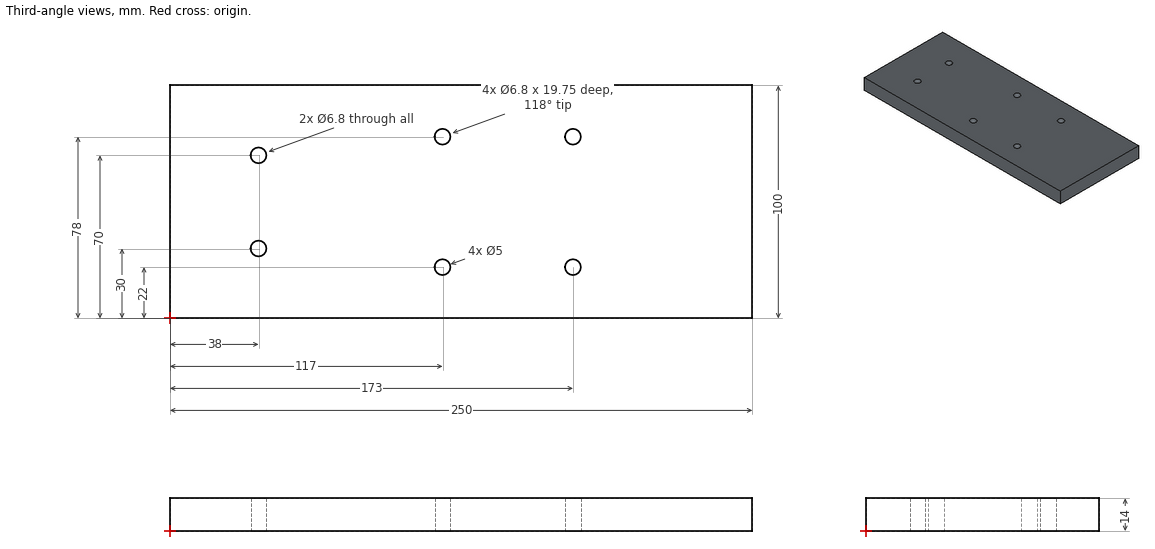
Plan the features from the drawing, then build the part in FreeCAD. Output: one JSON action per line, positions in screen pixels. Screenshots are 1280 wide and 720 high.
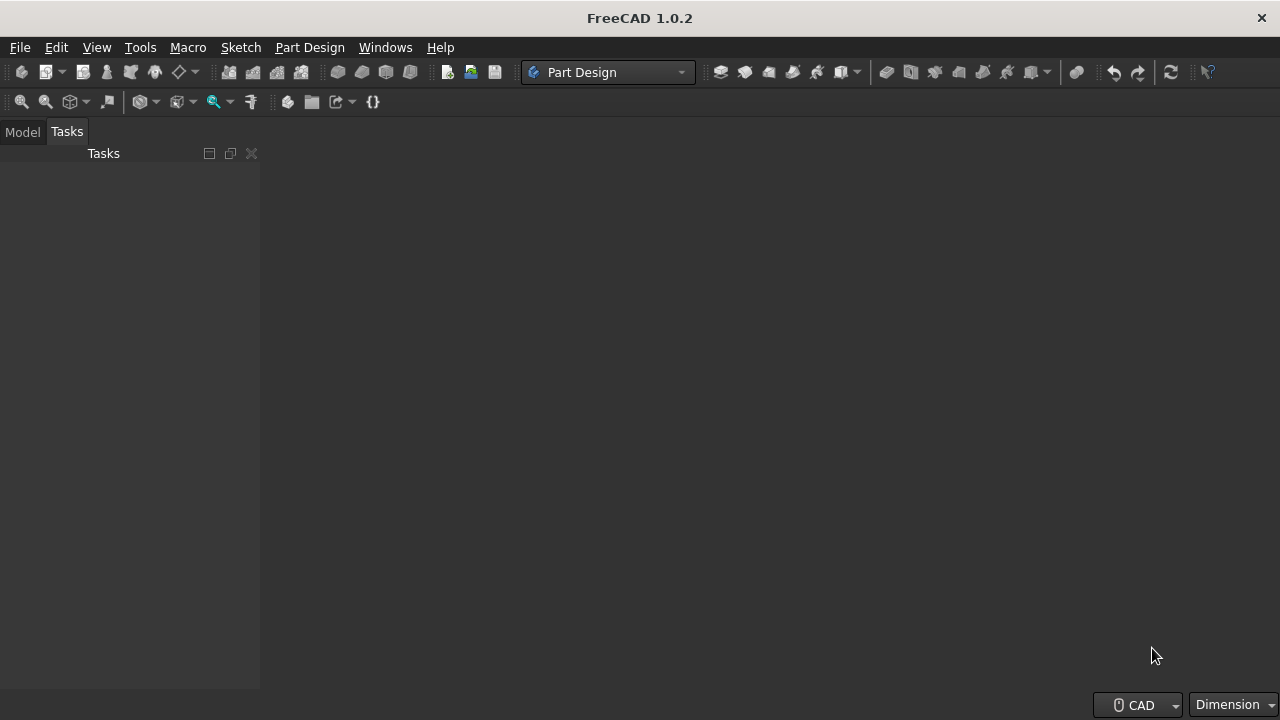
{"action": "left_click", "coordinate": [448, 72]}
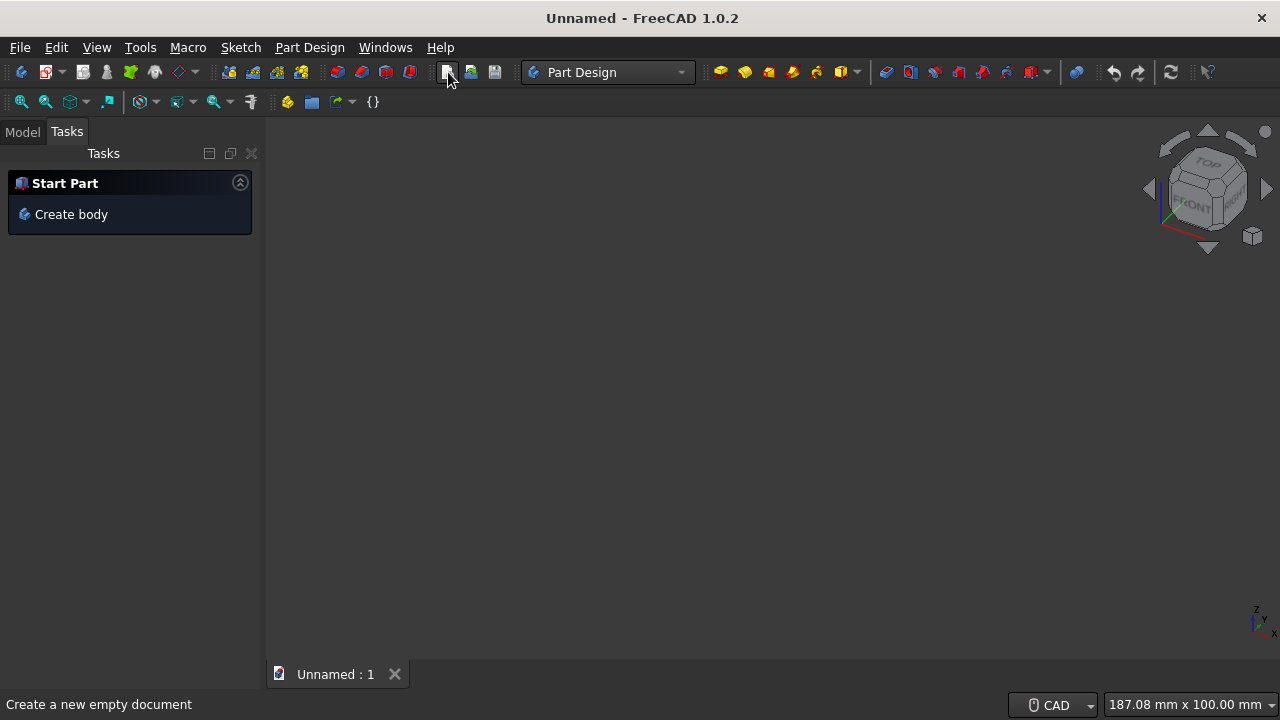
{"action": "left_click", "coordinate": [46, 72]}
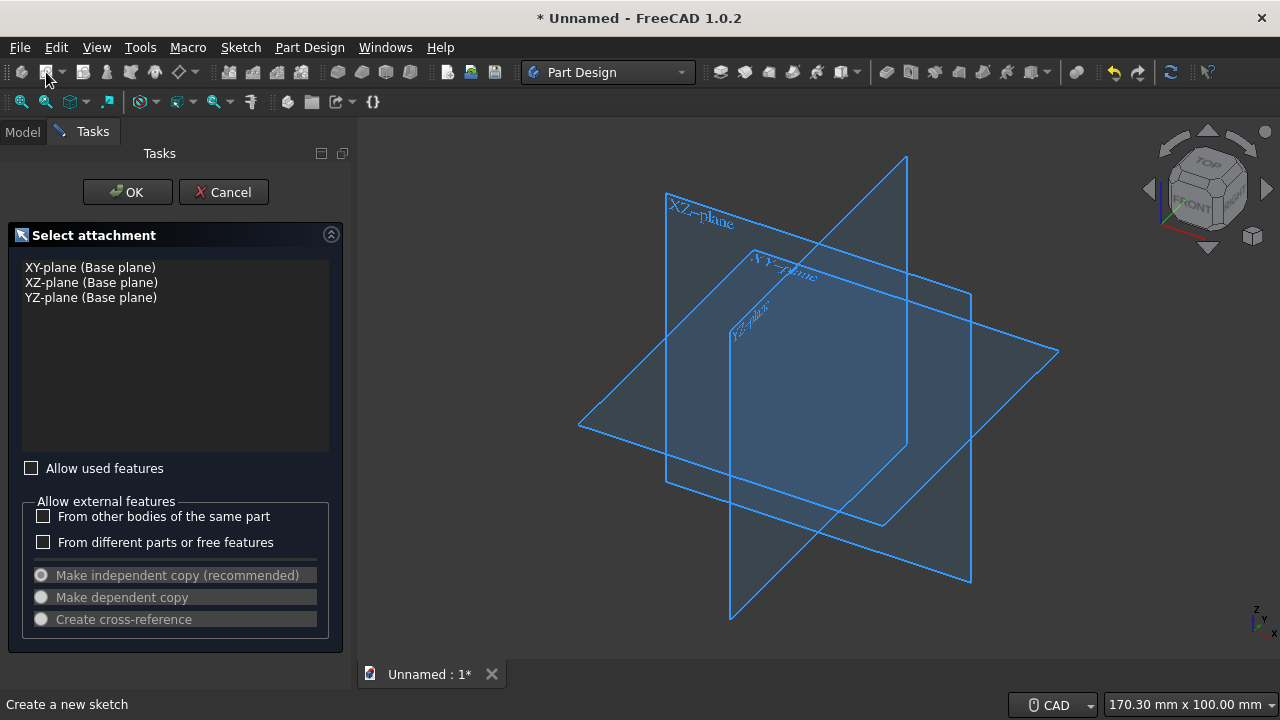
{"action": "left_click", "coordinate": [82, 268]}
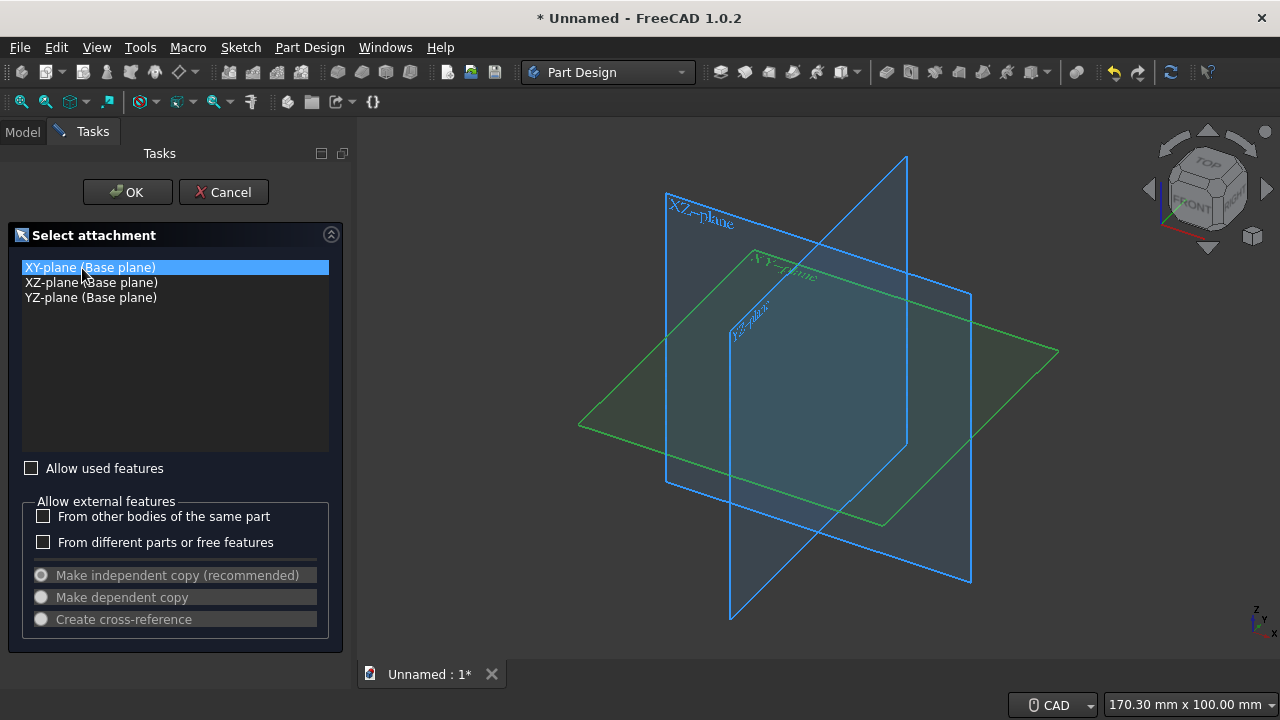
{"action": "left_click", "coordinate": [128, 192]}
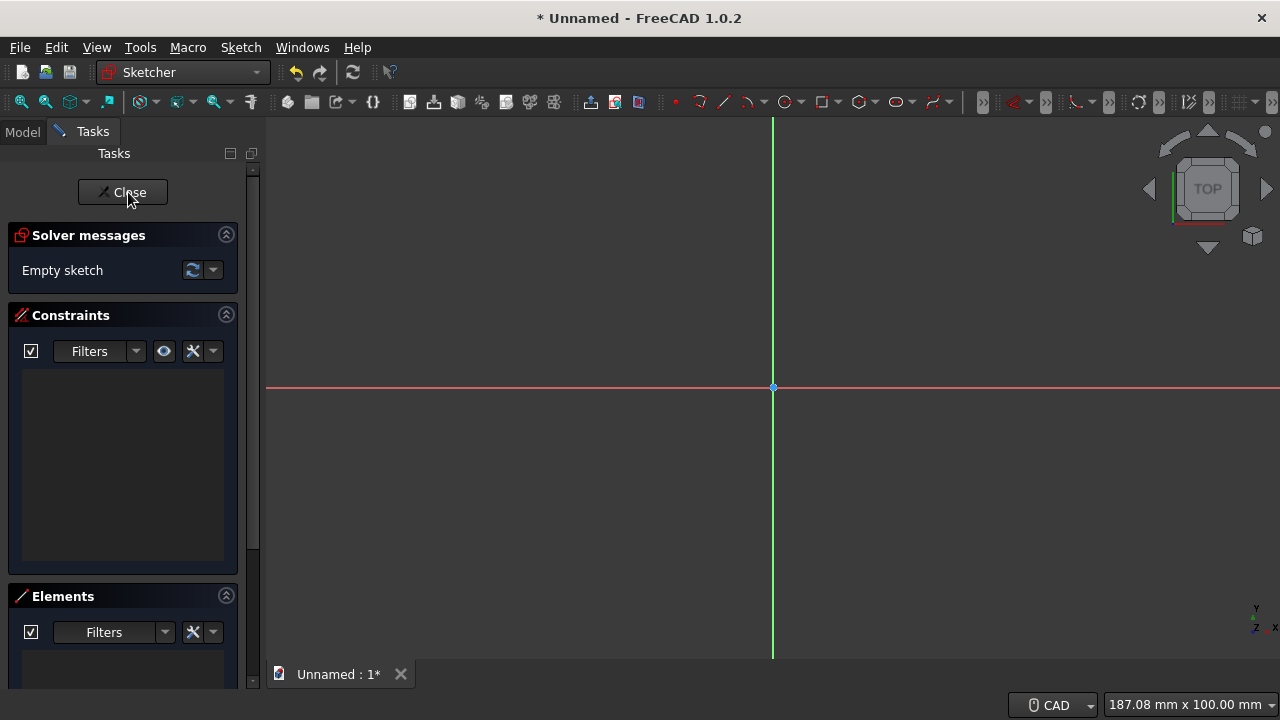
{"action": "scroll", "coordinate": [294, 546], "scroll_direction": "down", "scroll_amount": 5}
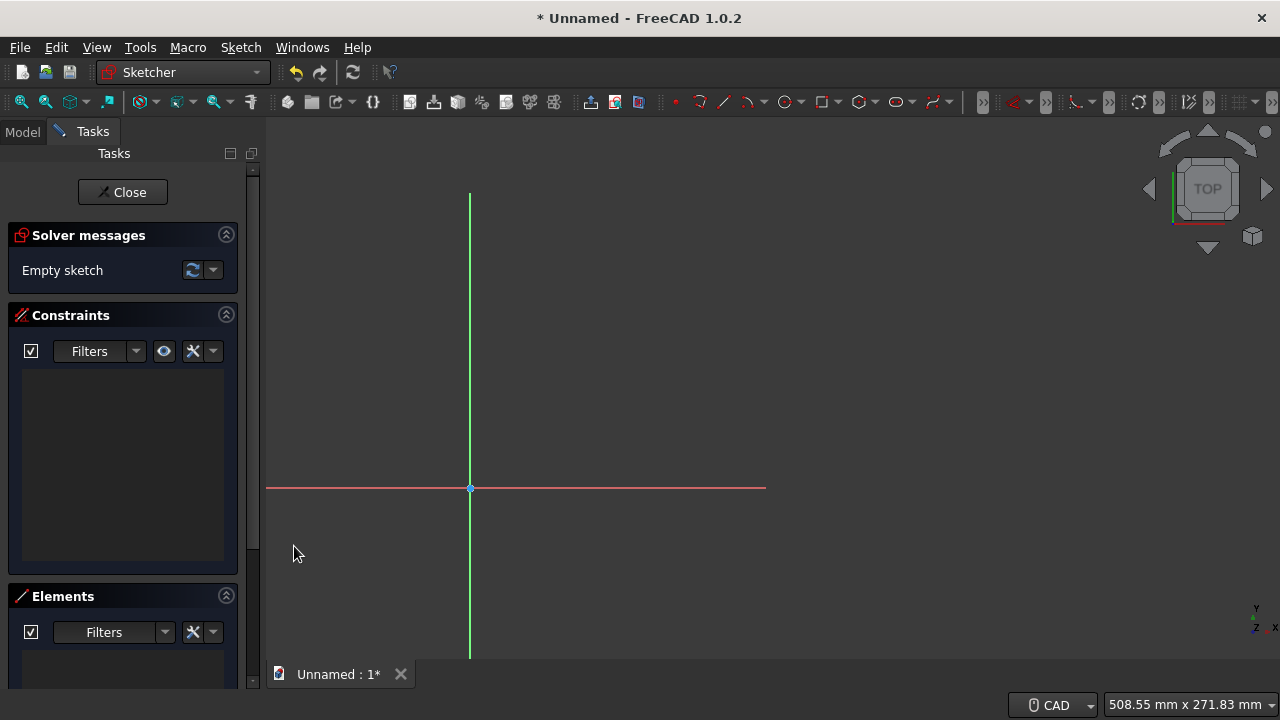
{"action": "left_click", "coordinate": [822, 102]}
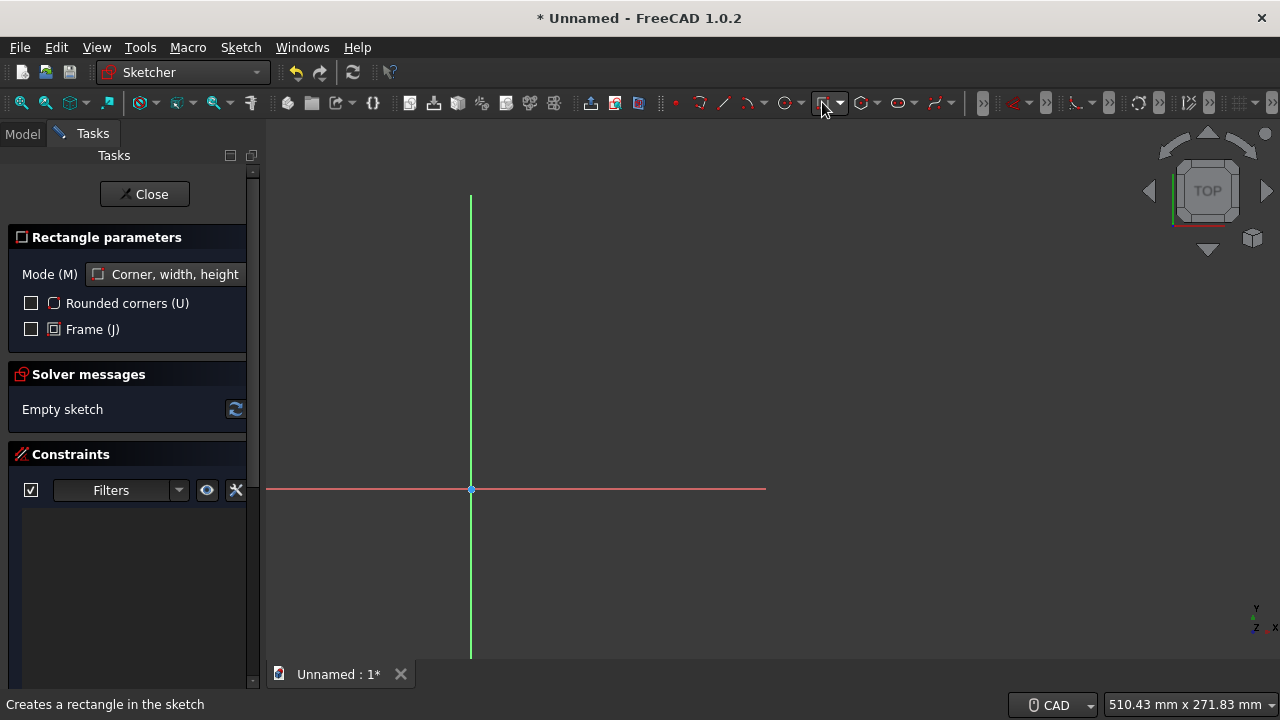
{"action": "left_click", "coordinate": [471, 489]}
{"action": "left_click", "coordinate": [968, 290]}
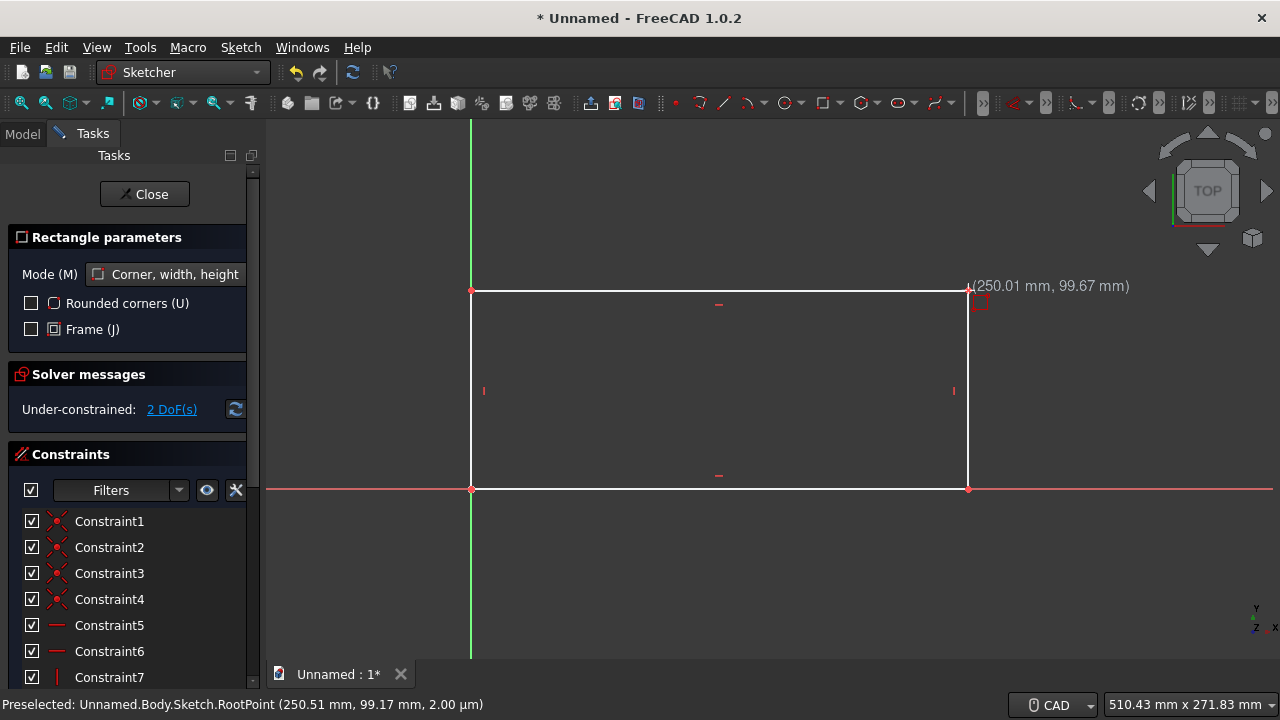
{"action": "key", "text": "g c"}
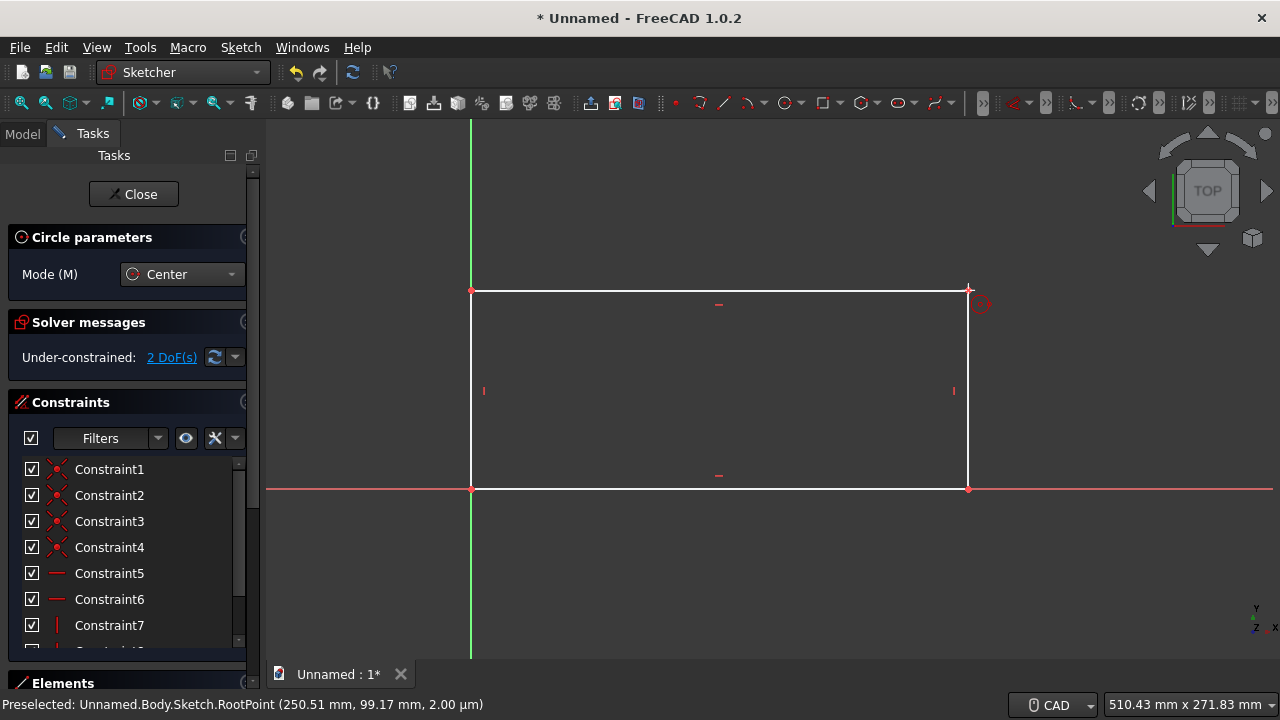
{"action": "scroll", "coordinate": [704, 445], "scroll_direction": "up", "scroll_amount": 8}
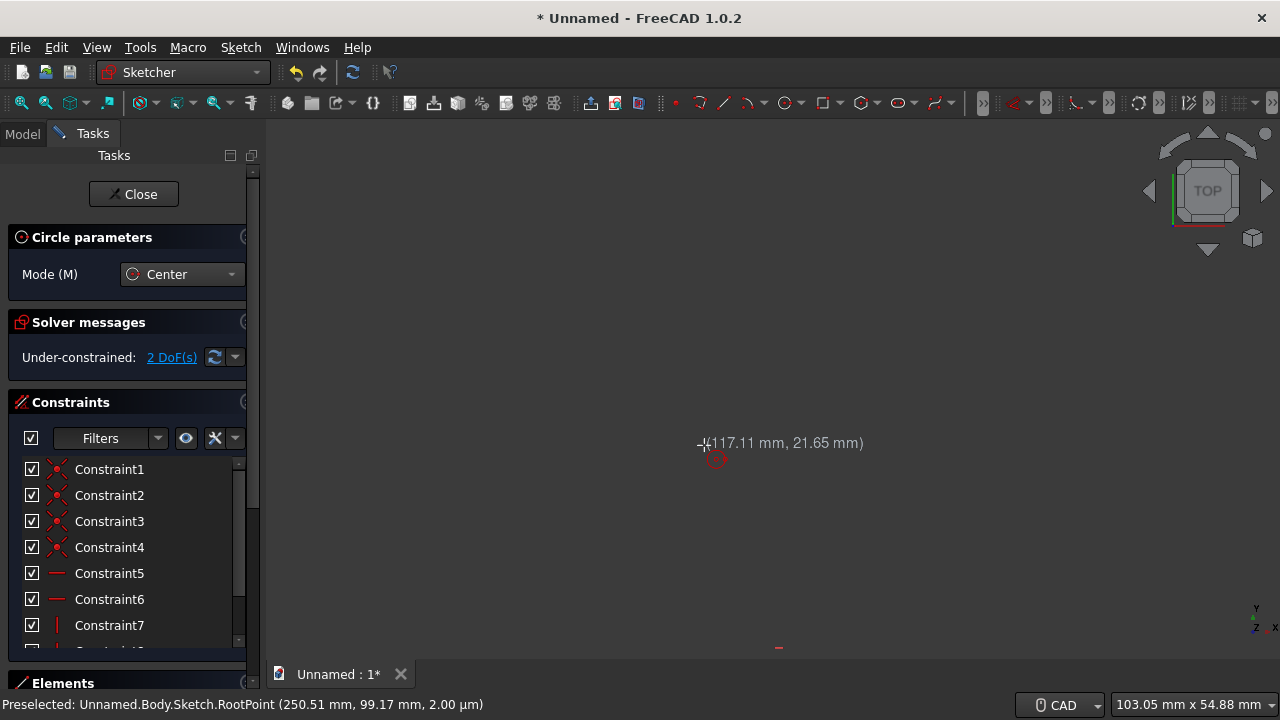
{"action": "scroll", "coordinate": [680, 461], "scroll_direction": "down", "scroll_amount": 7}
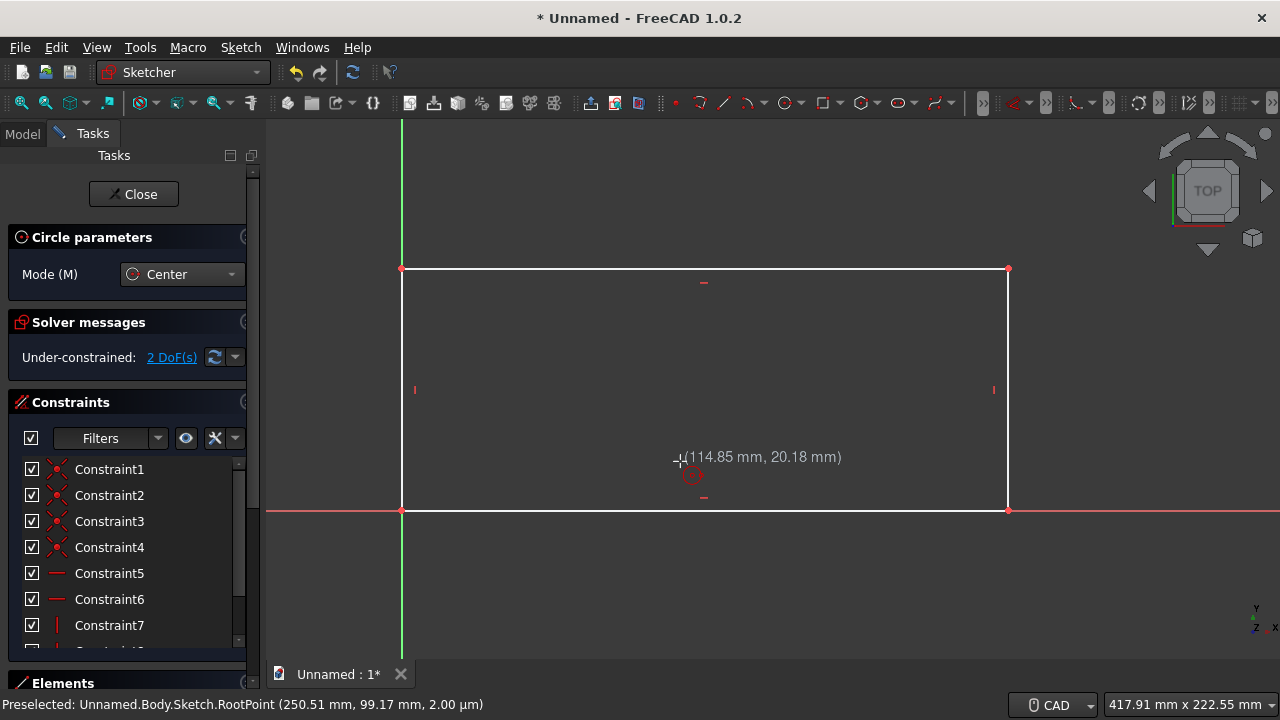
{"action": "left_click", "coordinate": [686, 457]}